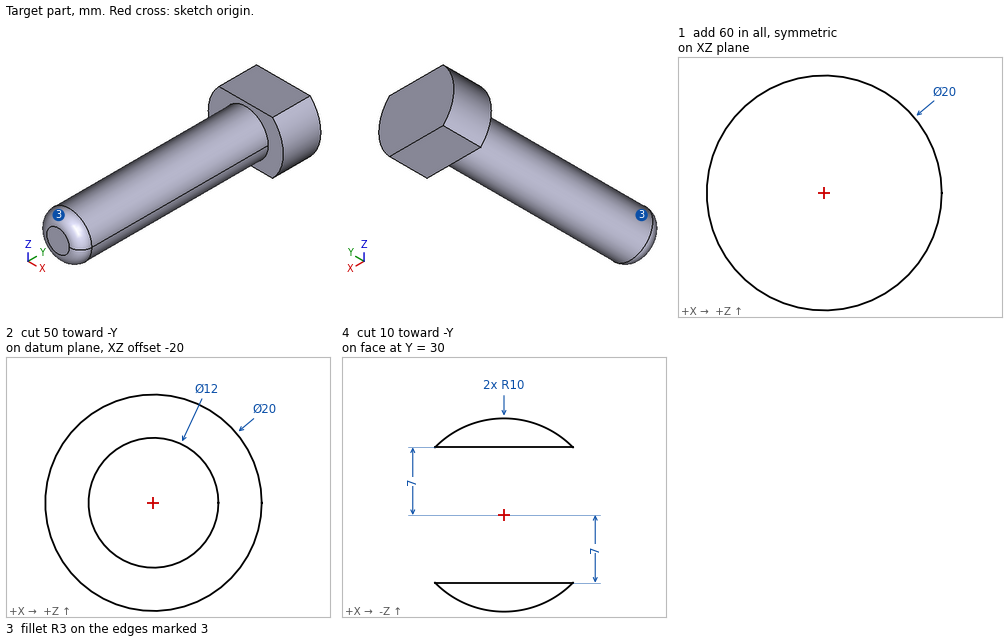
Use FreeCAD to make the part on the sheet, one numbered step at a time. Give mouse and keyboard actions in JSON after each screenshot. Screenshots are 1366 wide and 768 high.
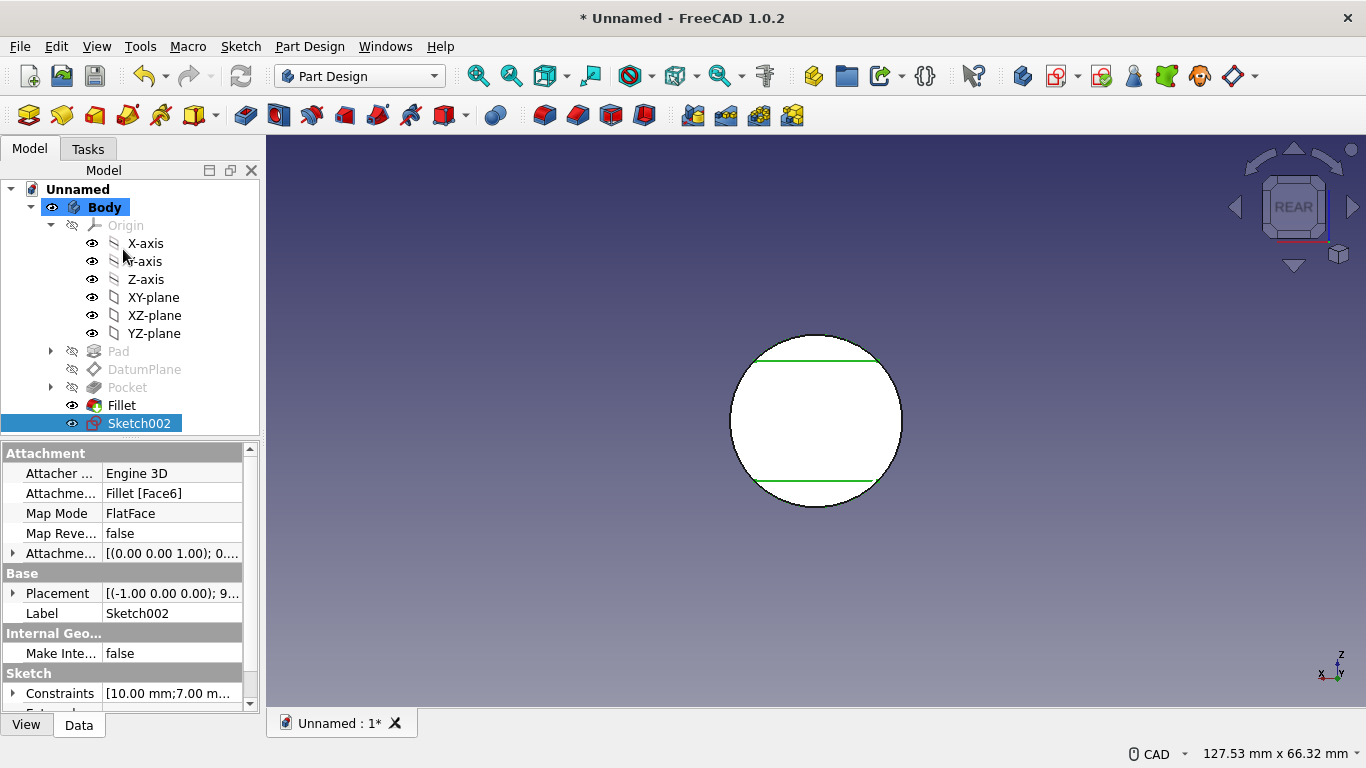
{"action": "left_click", "coordinate": [246, 116]}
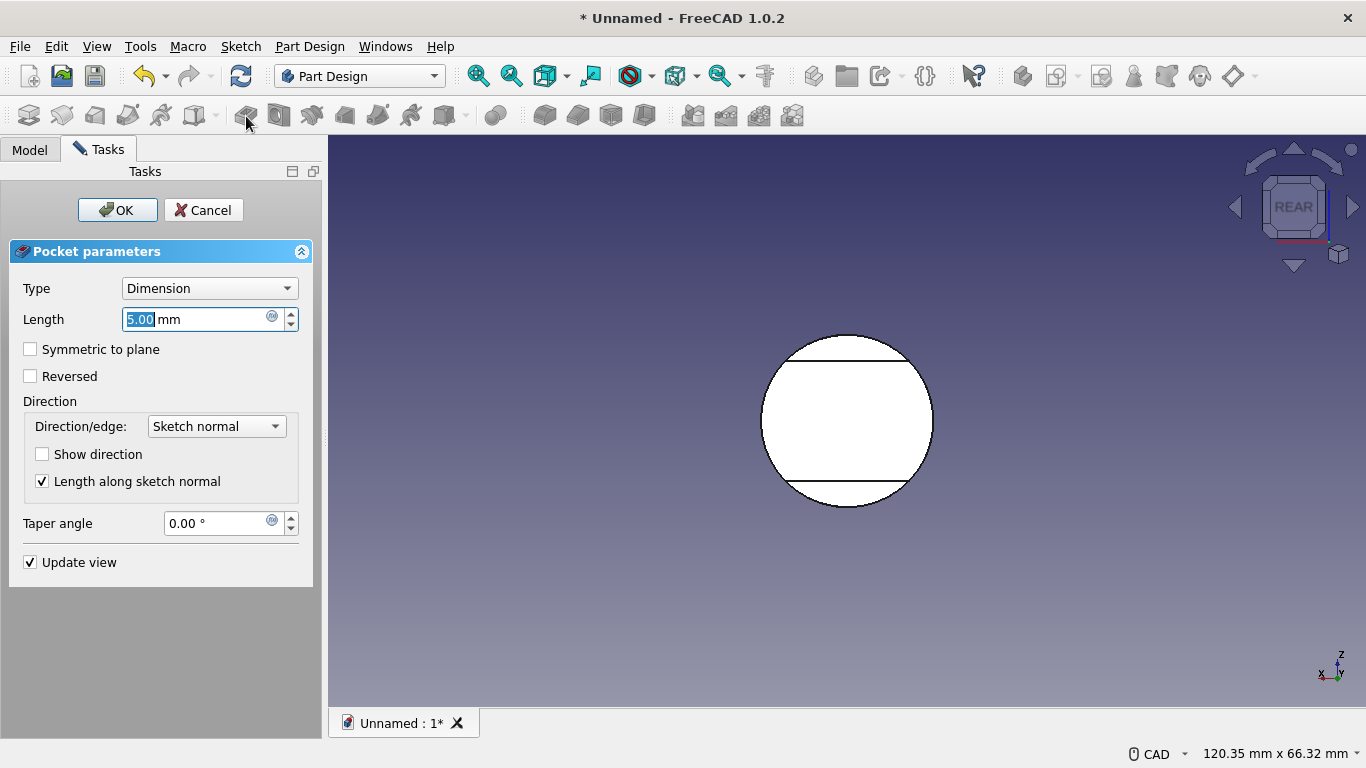
{"action": "type", "text": "10"}
{"action": "key", "text": "Tab"}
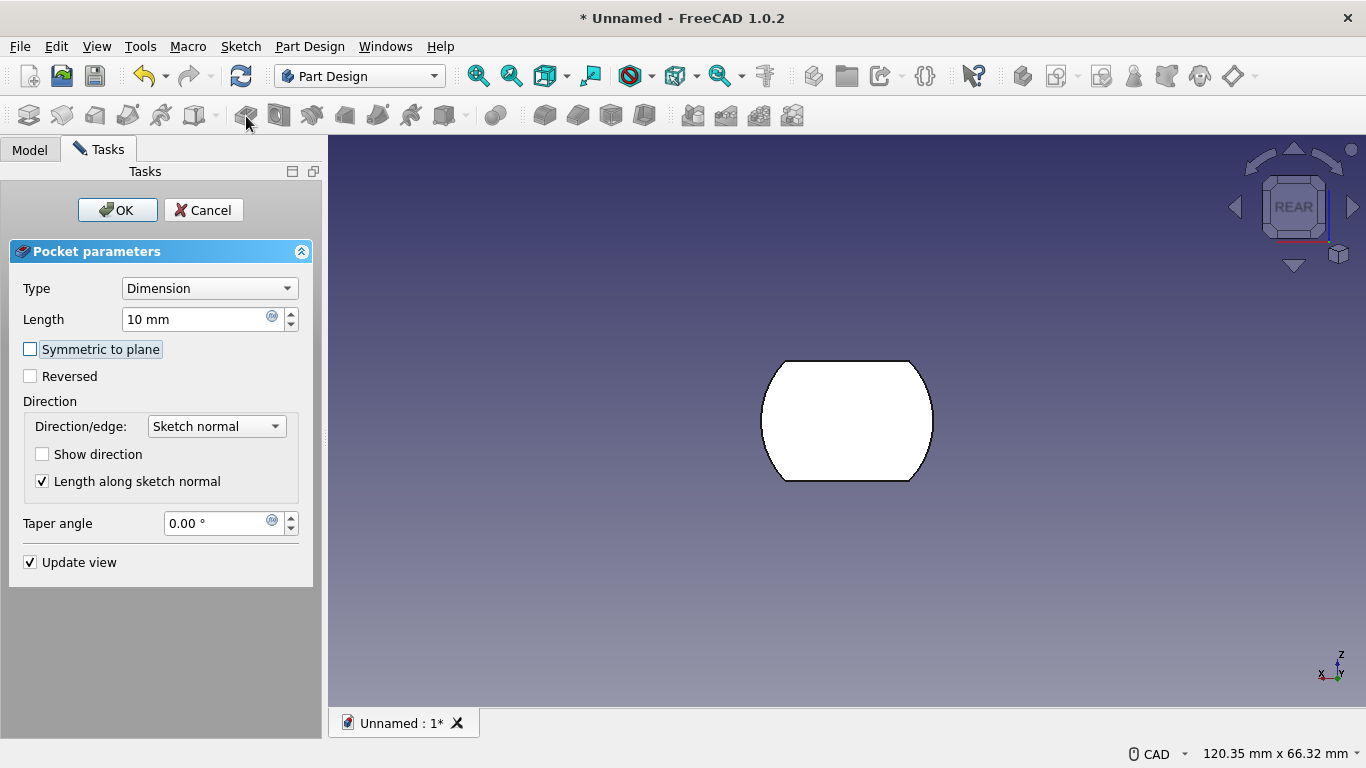
{"action": "left_click", "coordinate": [118, 210]}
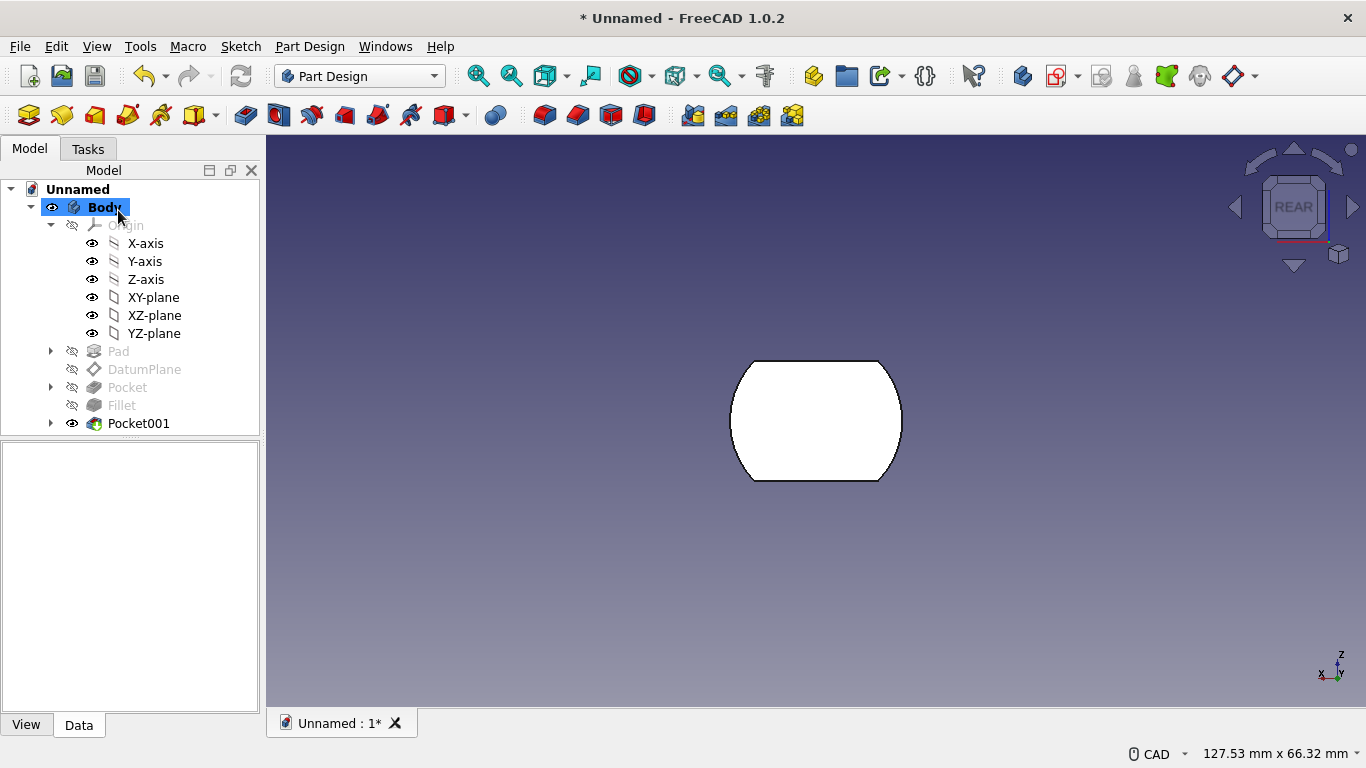
{"action": "key", "text": "0"}